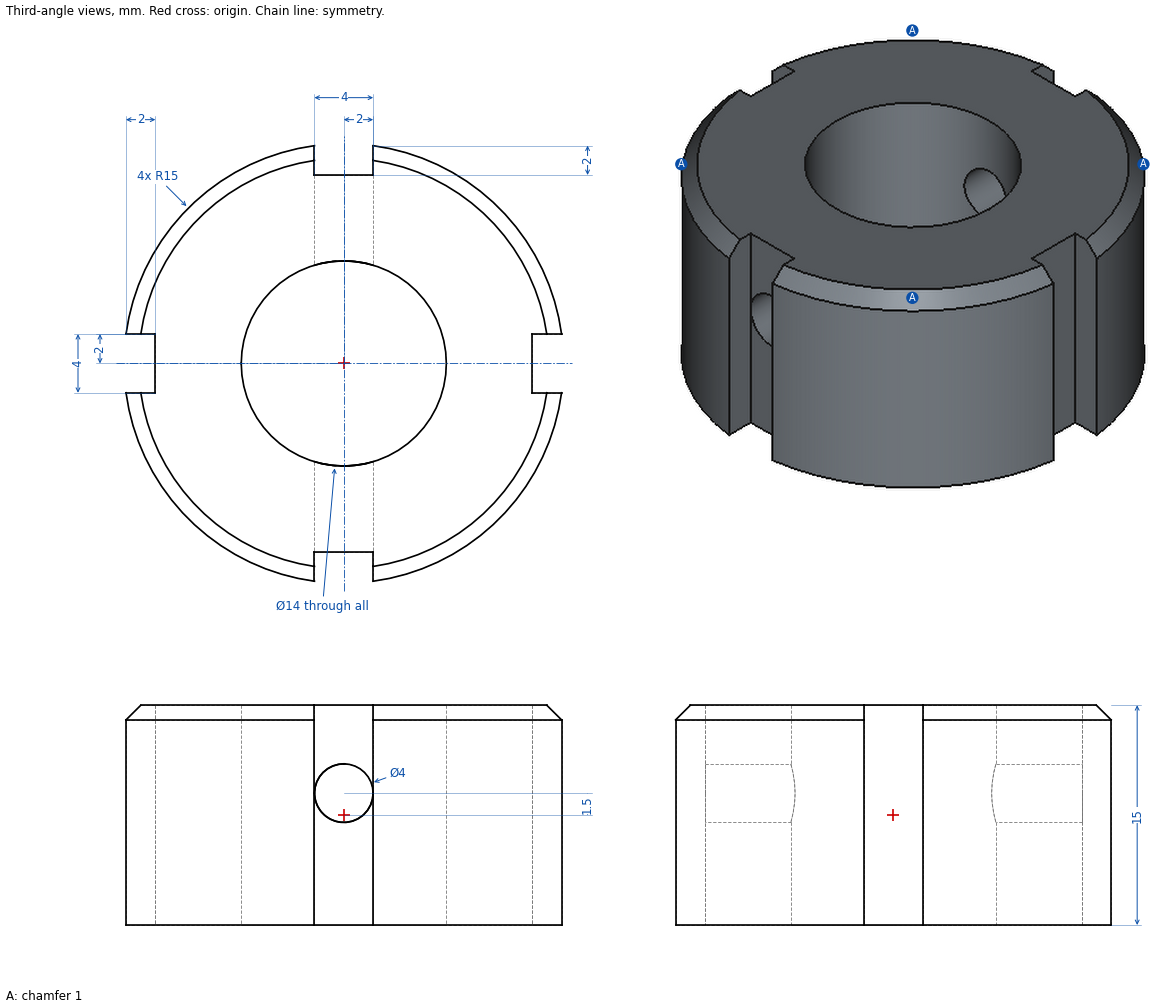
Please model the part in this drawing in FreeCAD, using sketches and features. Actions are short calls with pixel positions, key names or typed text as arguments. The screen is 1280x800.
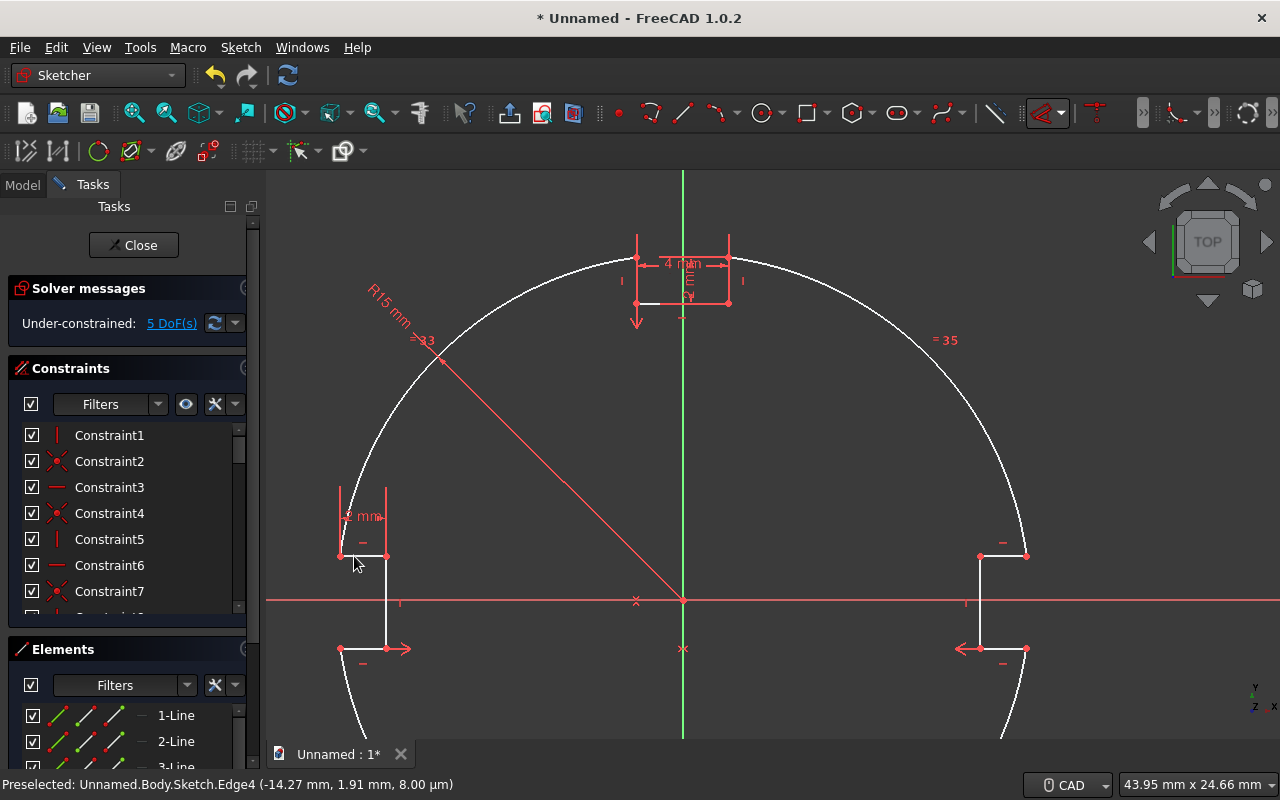
click(386, 584)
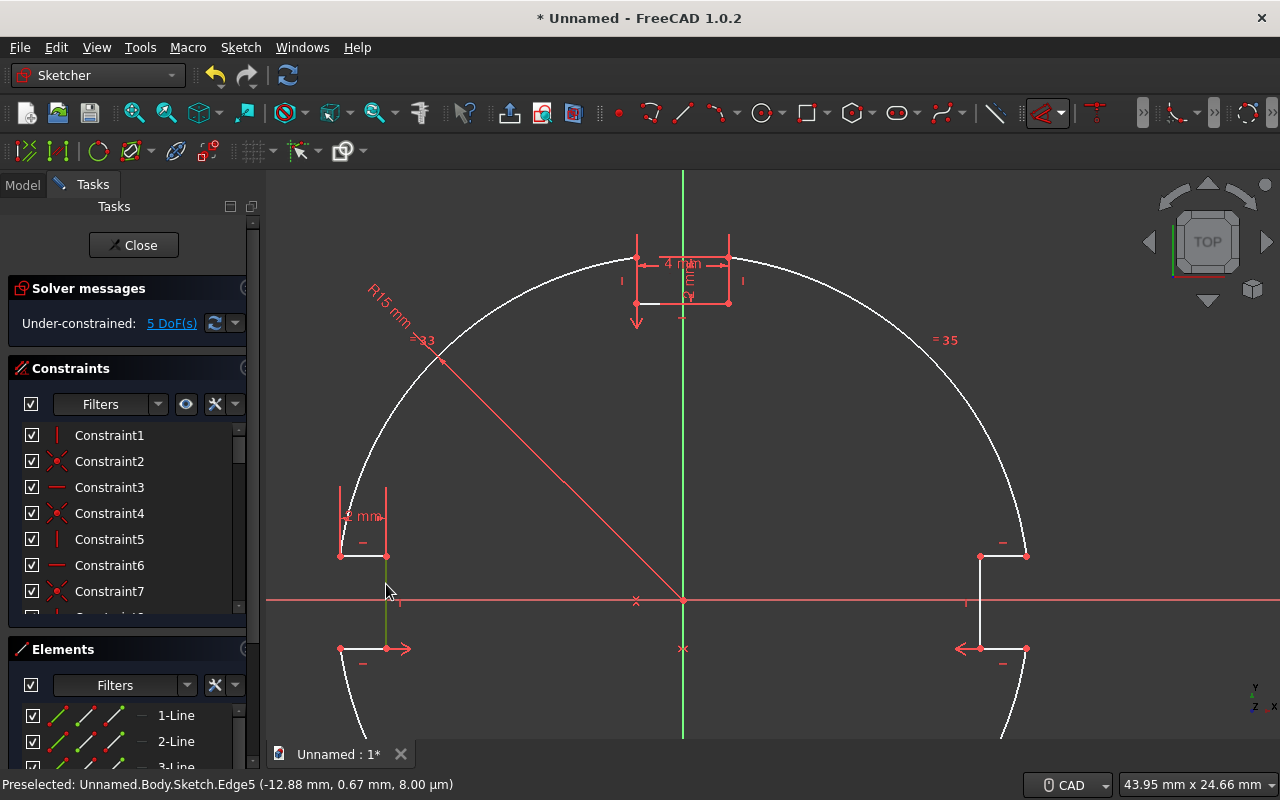
key(i)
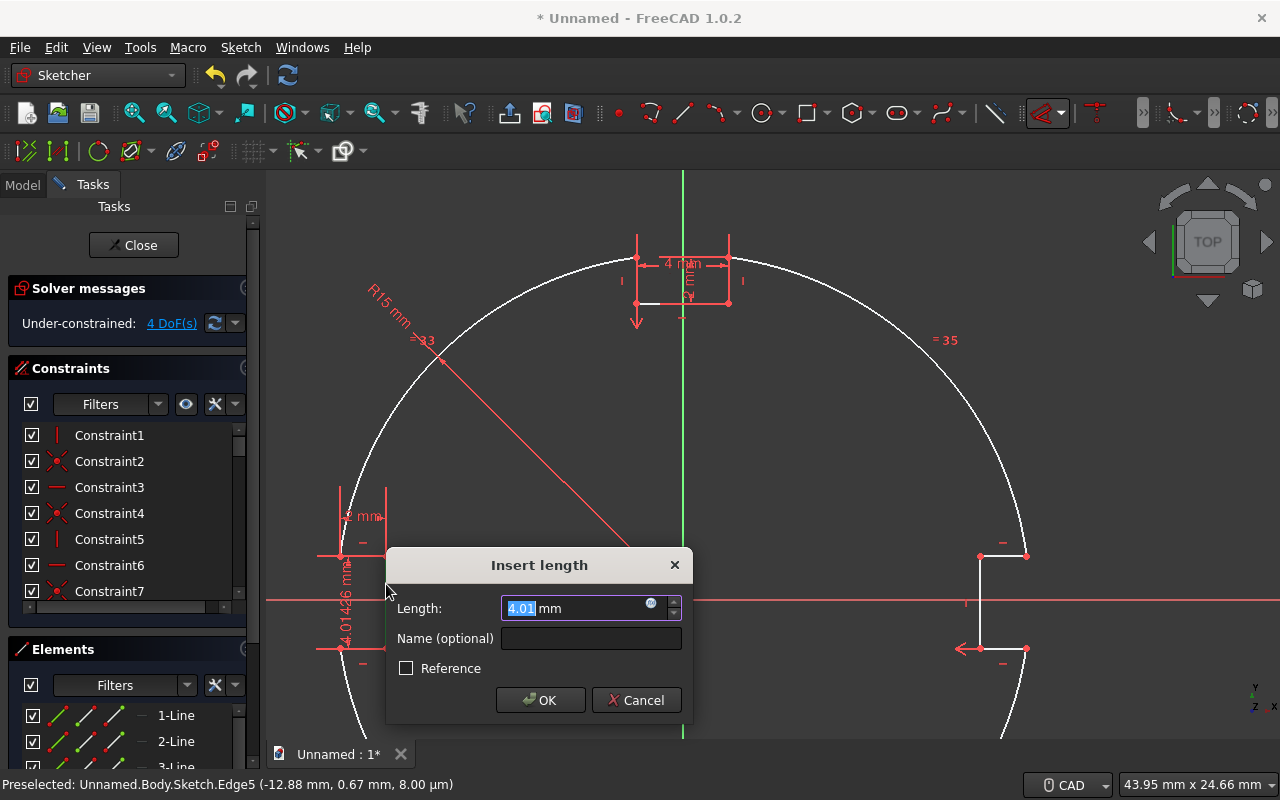
text(4)
key(Return)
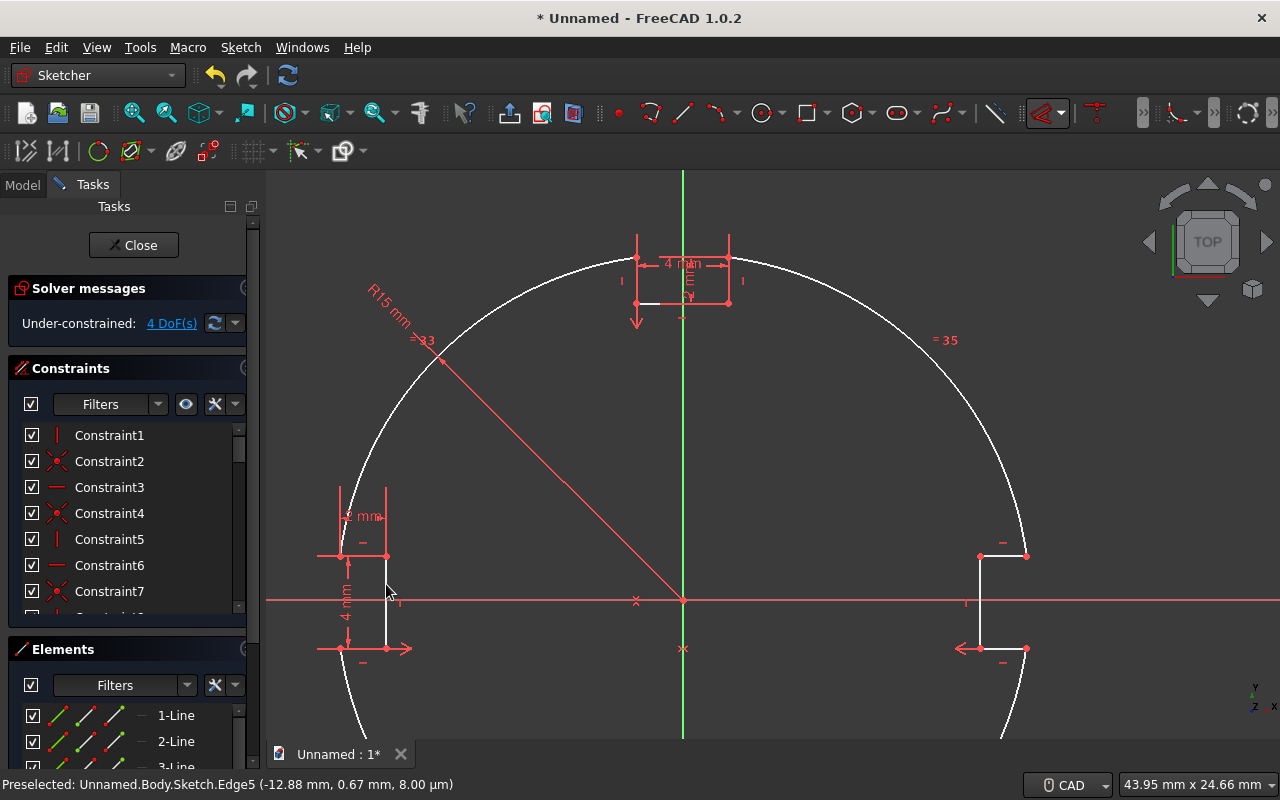
scroll(730, 277, down, 3)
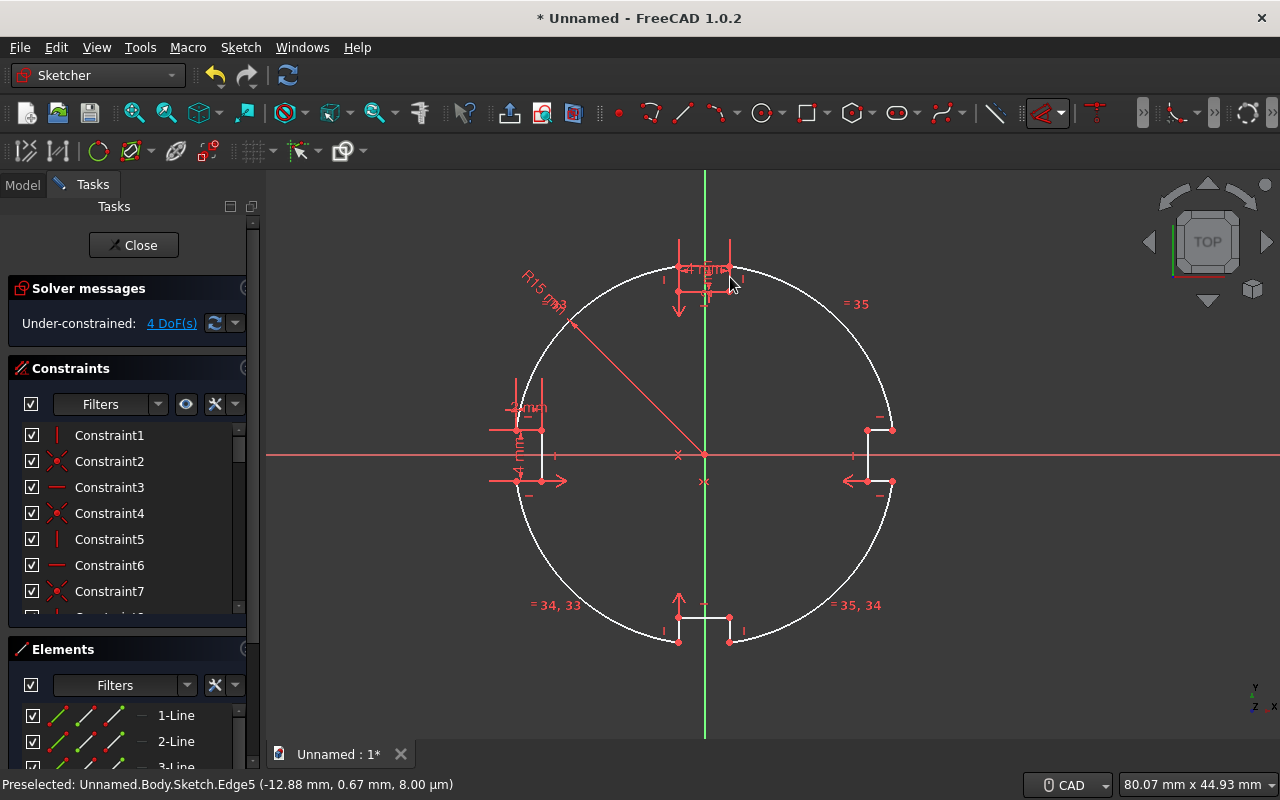
scroll(694, 618, up, 2)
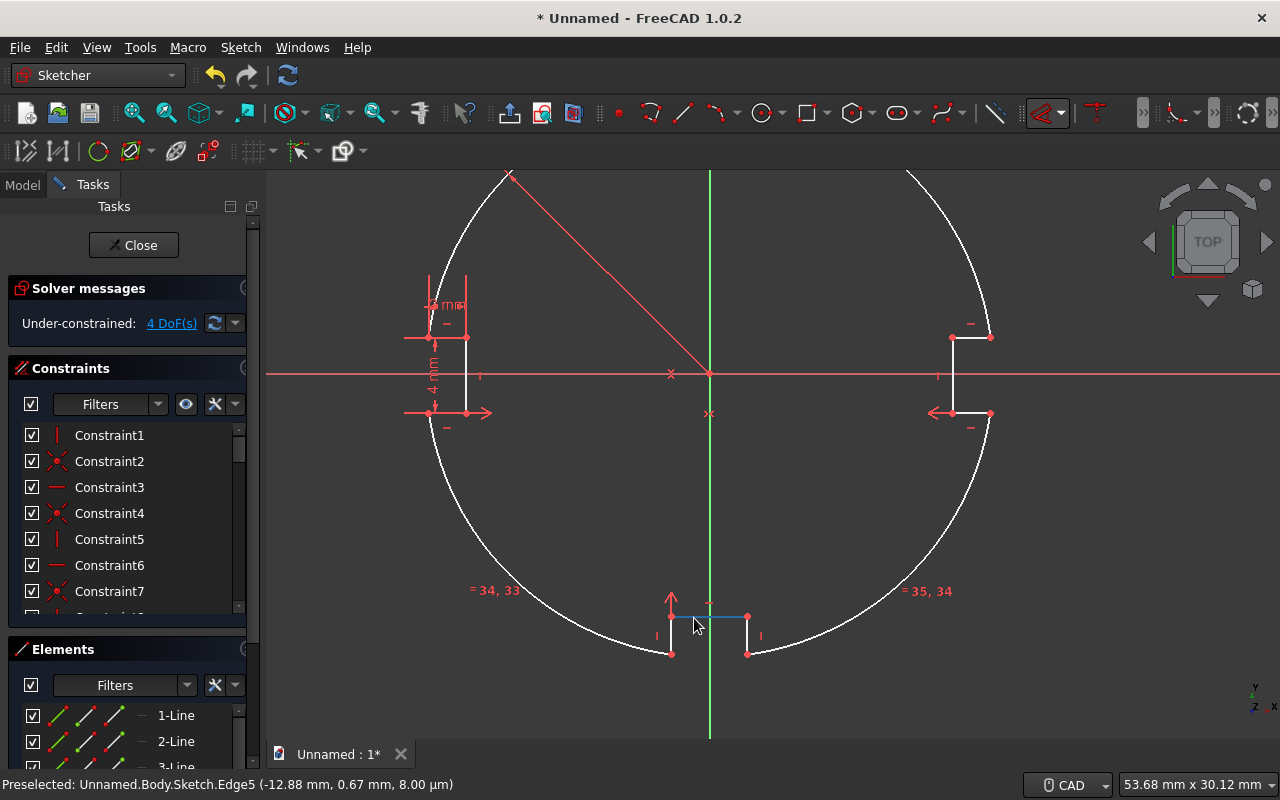
click(694, 617)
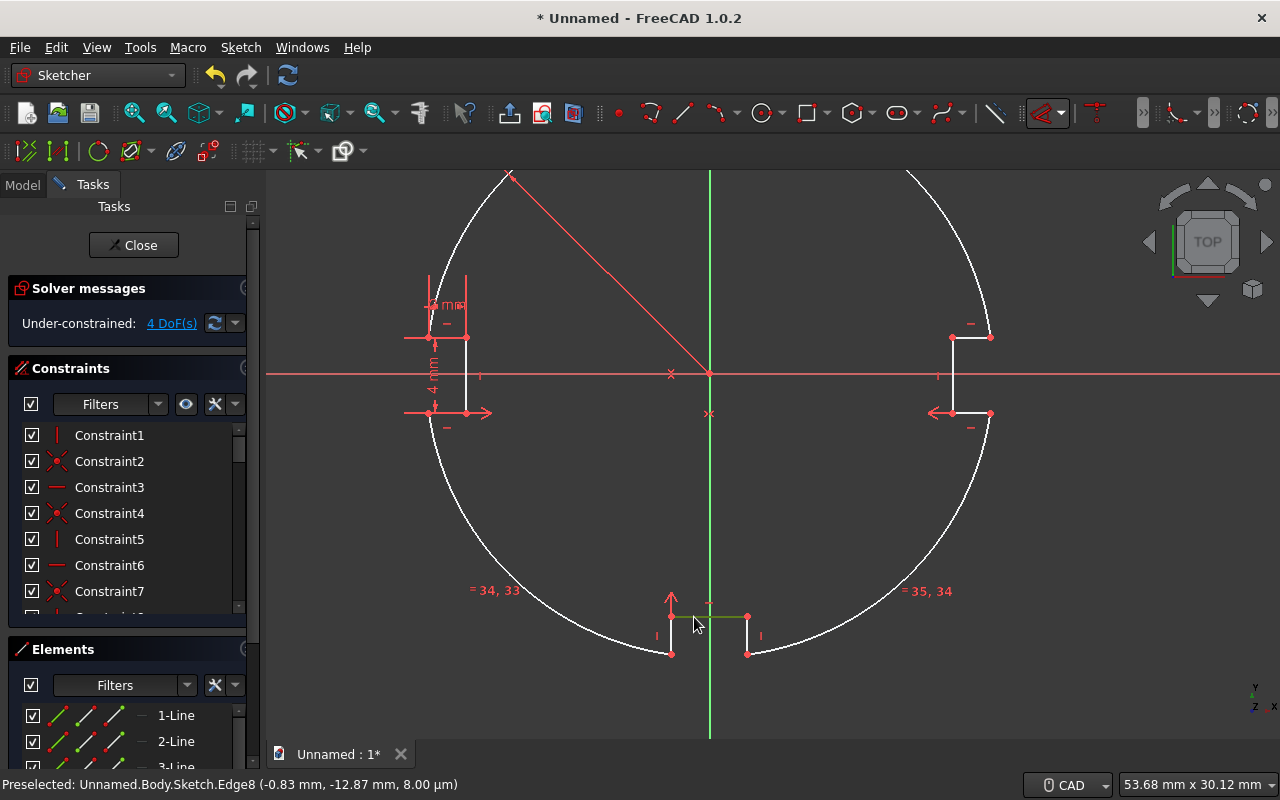
key(l)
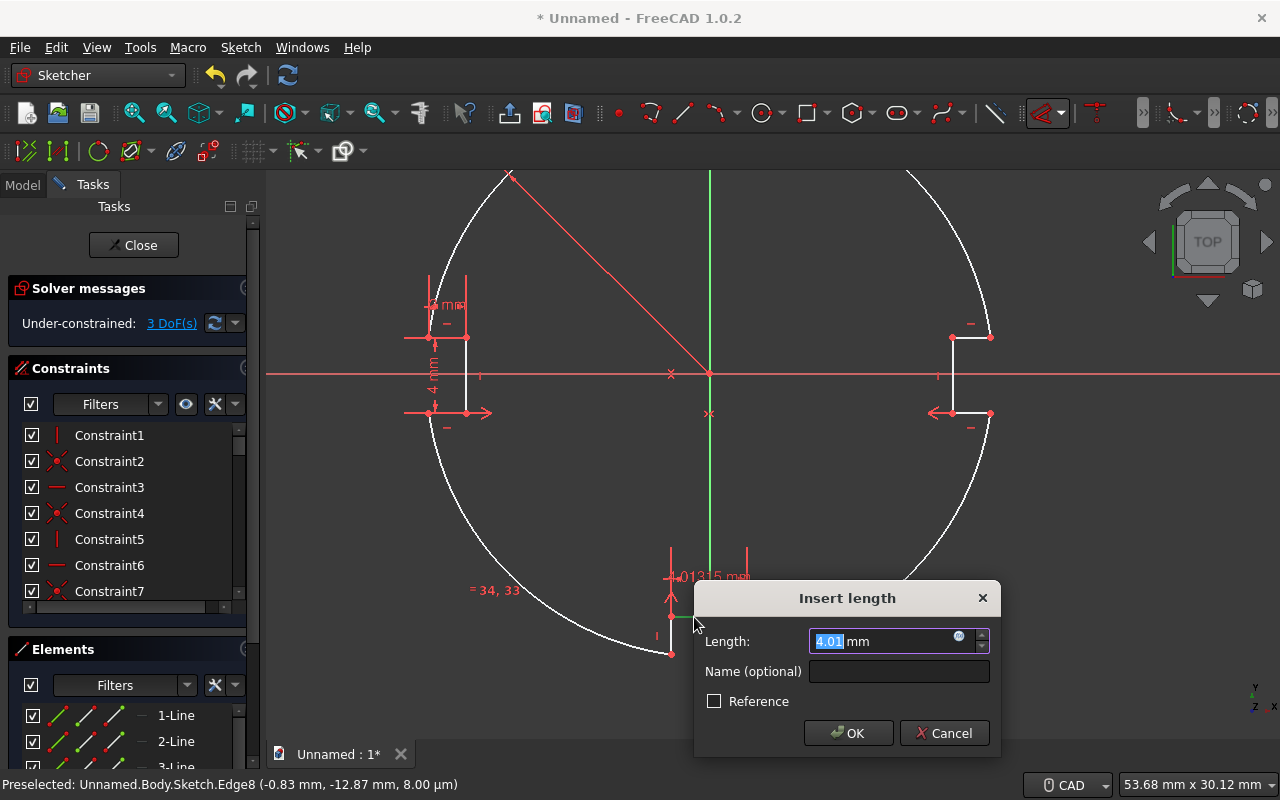
text(4)
key(Return)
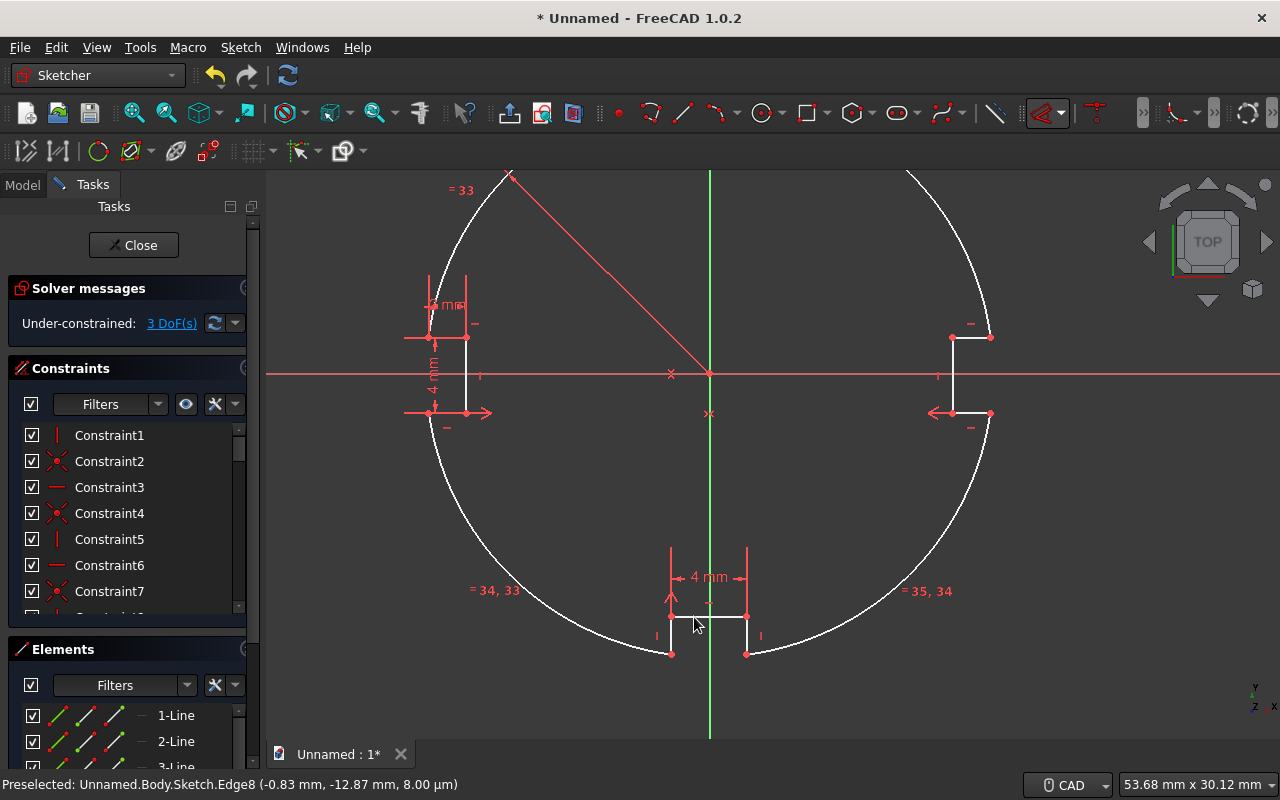
click(953, 391)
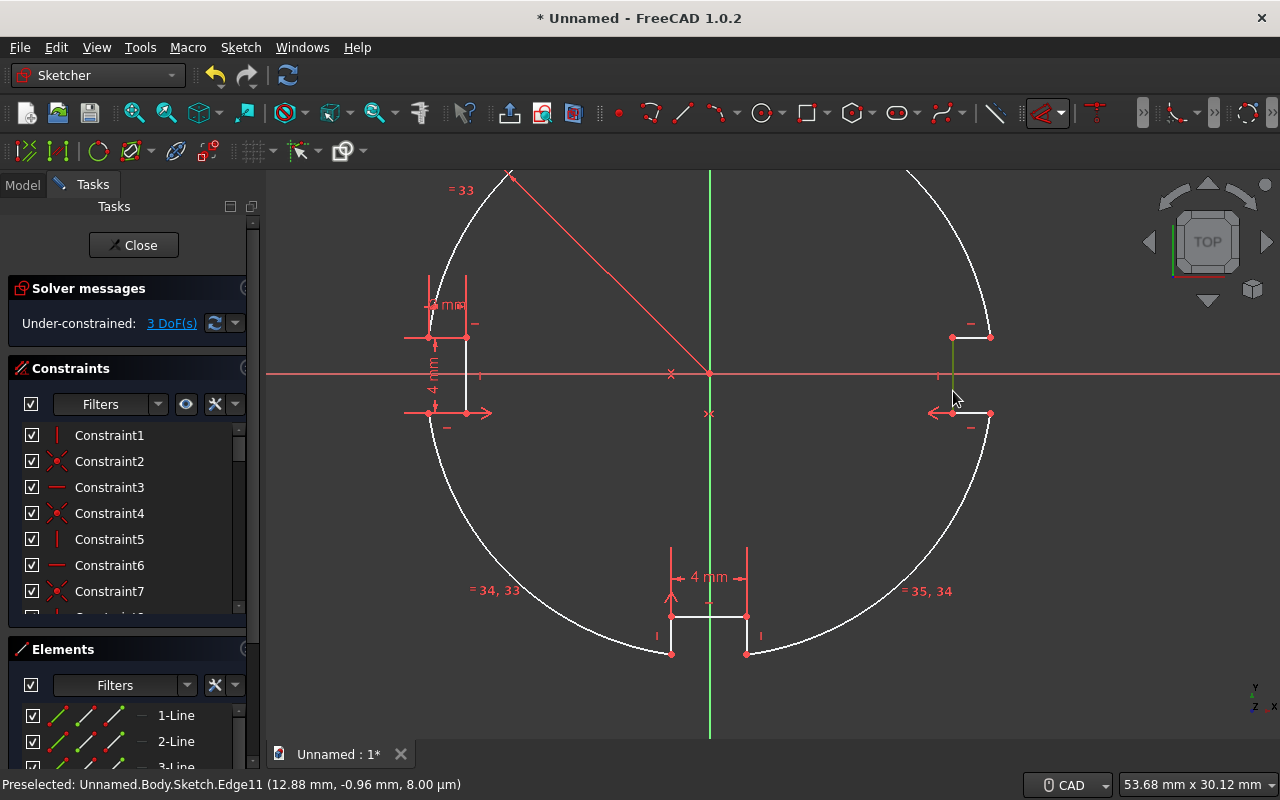
key(i)